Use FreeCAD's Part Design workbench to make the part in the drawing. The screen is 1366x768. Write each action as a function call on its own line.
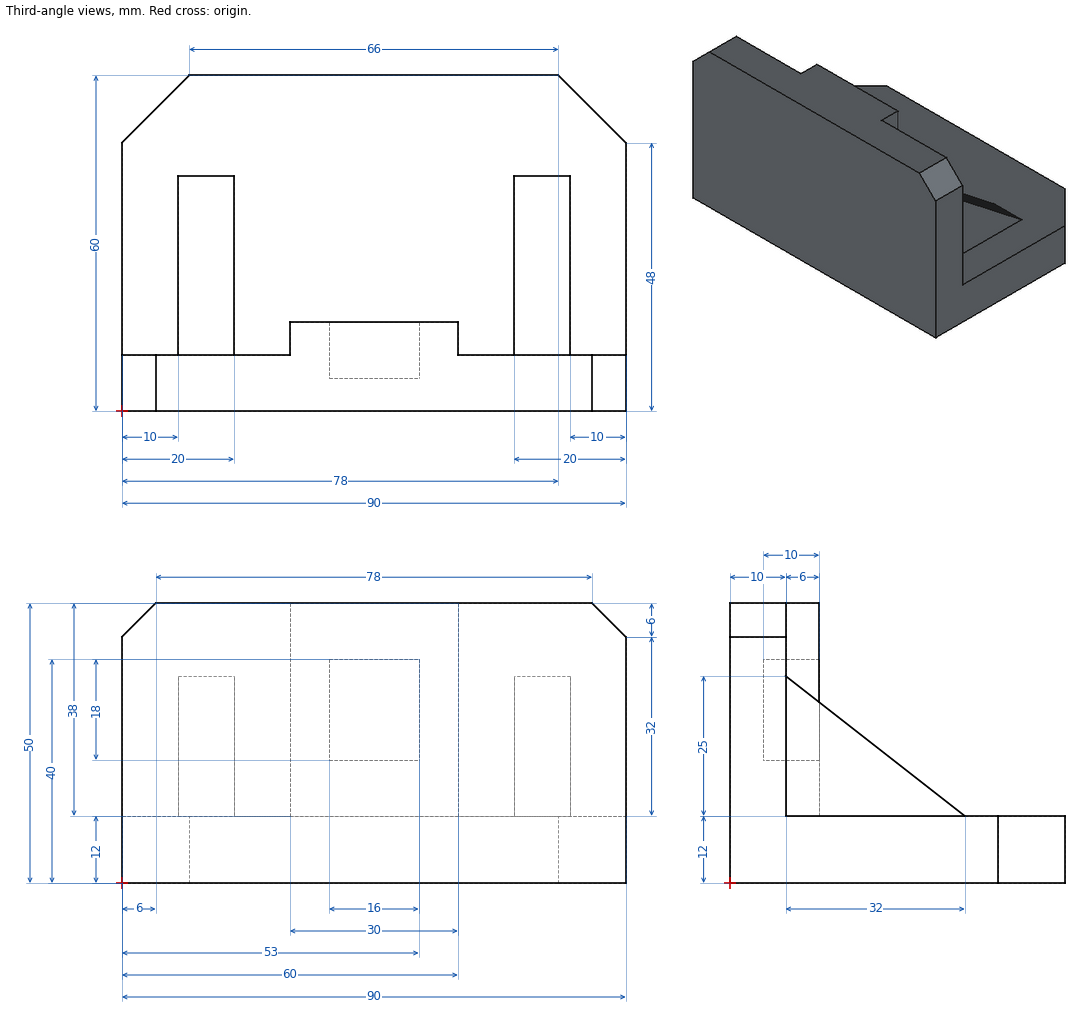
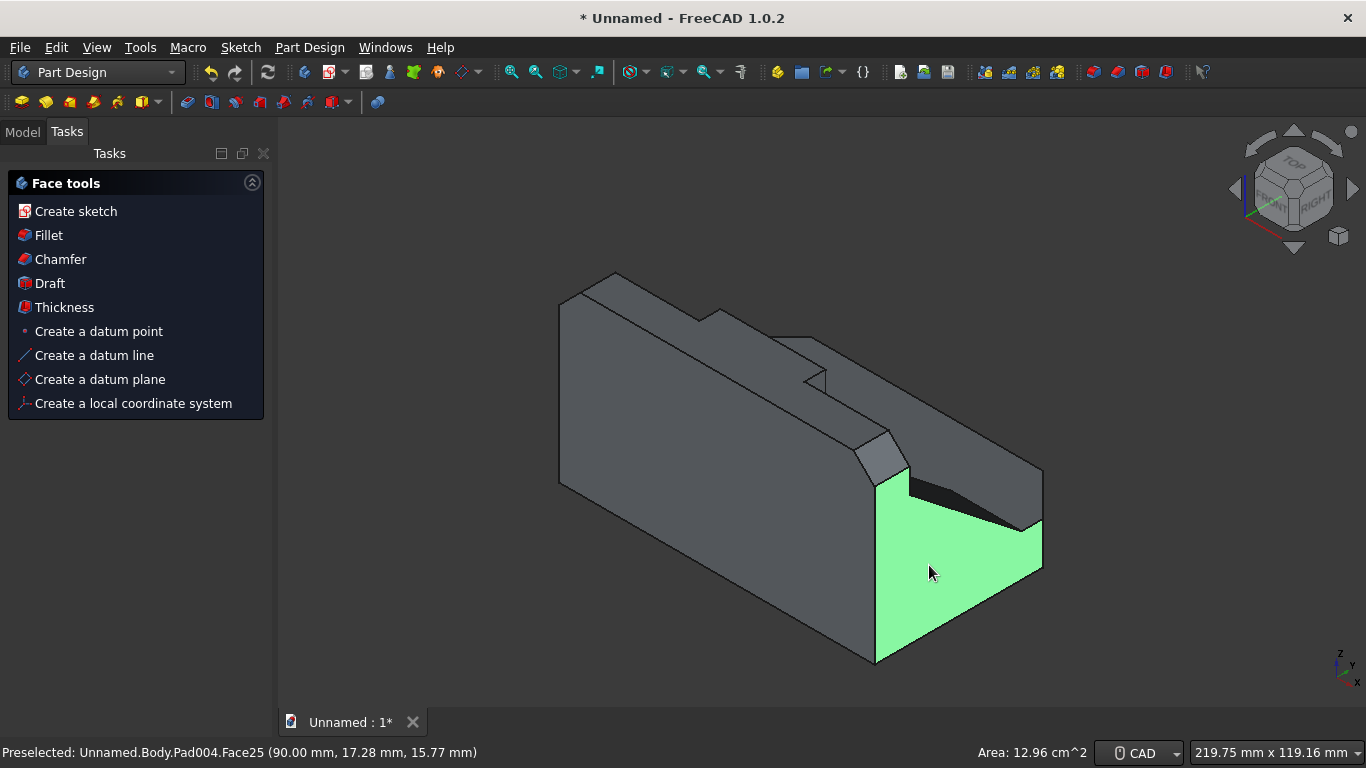
click(330, 72)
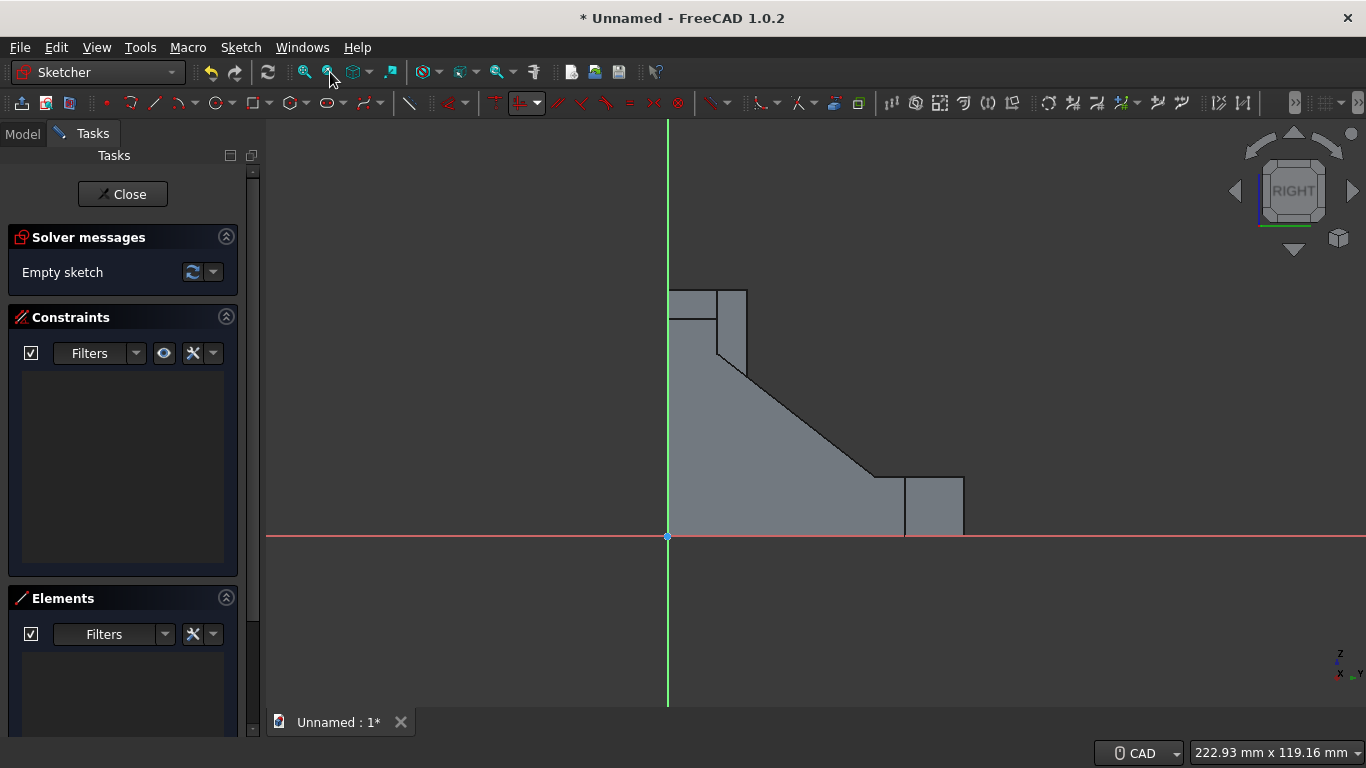
scroll(791, 471, up, 4)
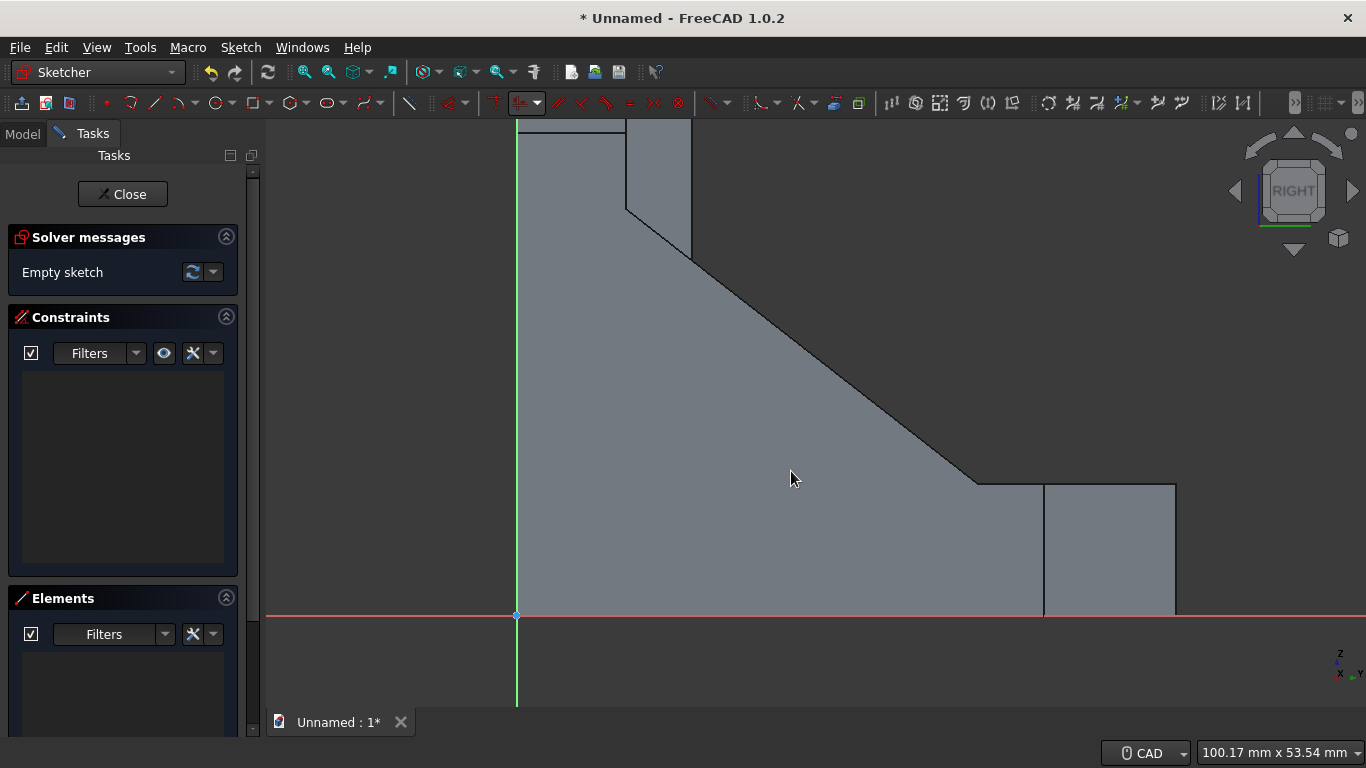
click(132, 104)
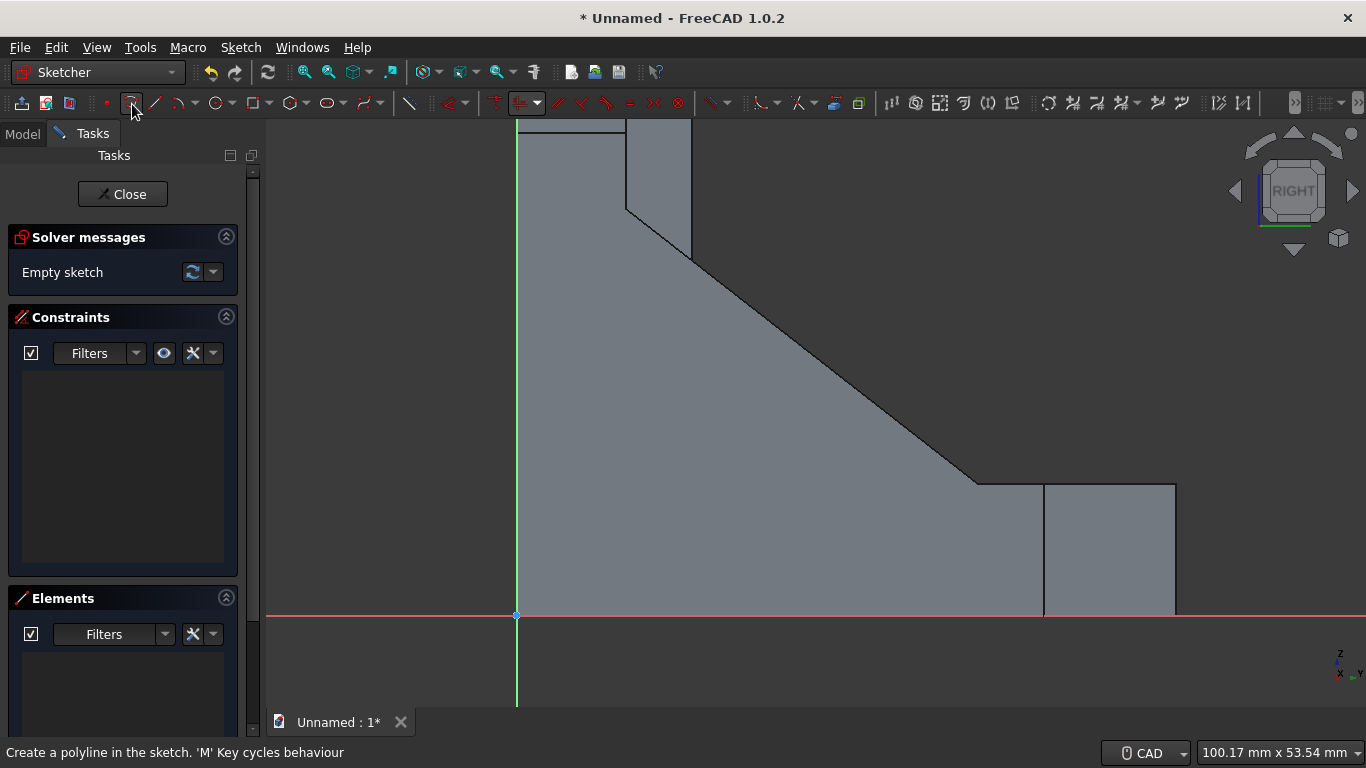
click(626, 484)
click(978, 484)
click(626, 209)
click(626, 485)
key(Escape)
key(Escape)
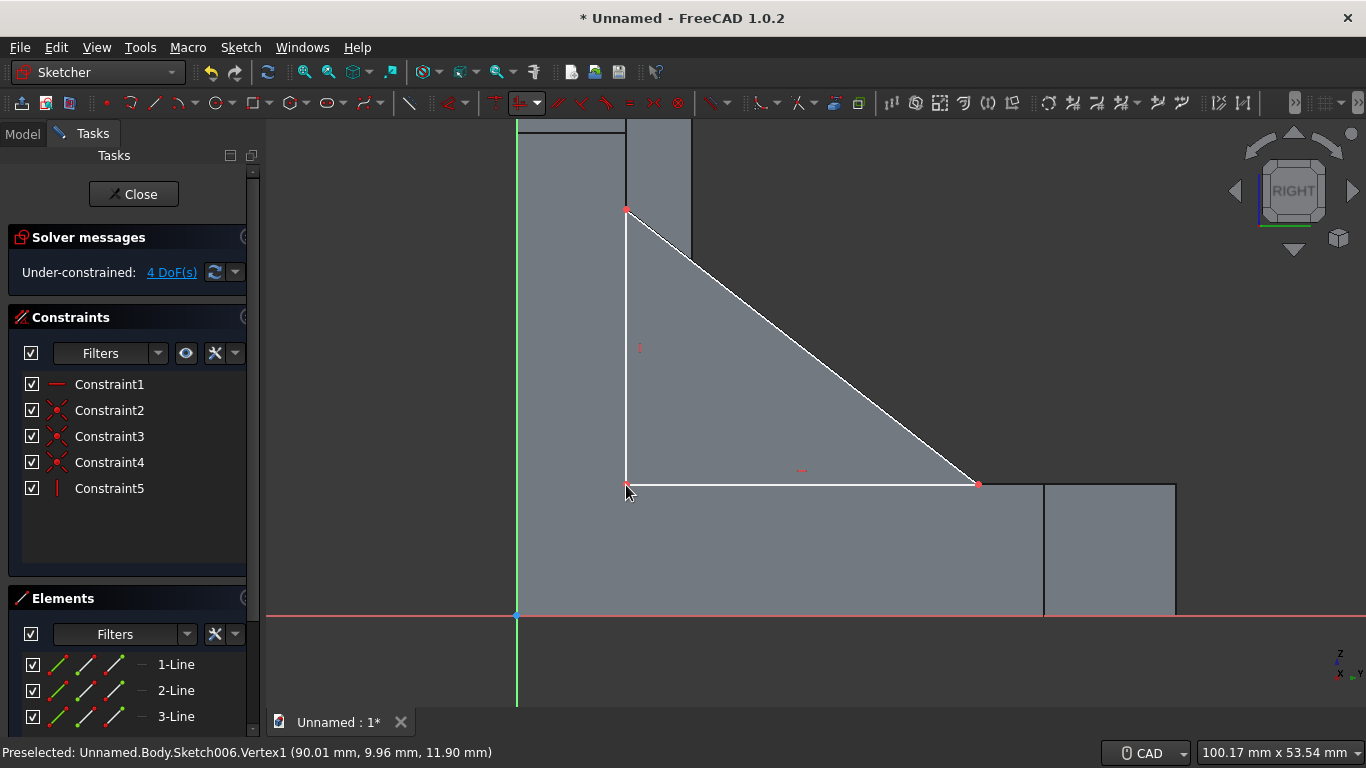
click(448, 104)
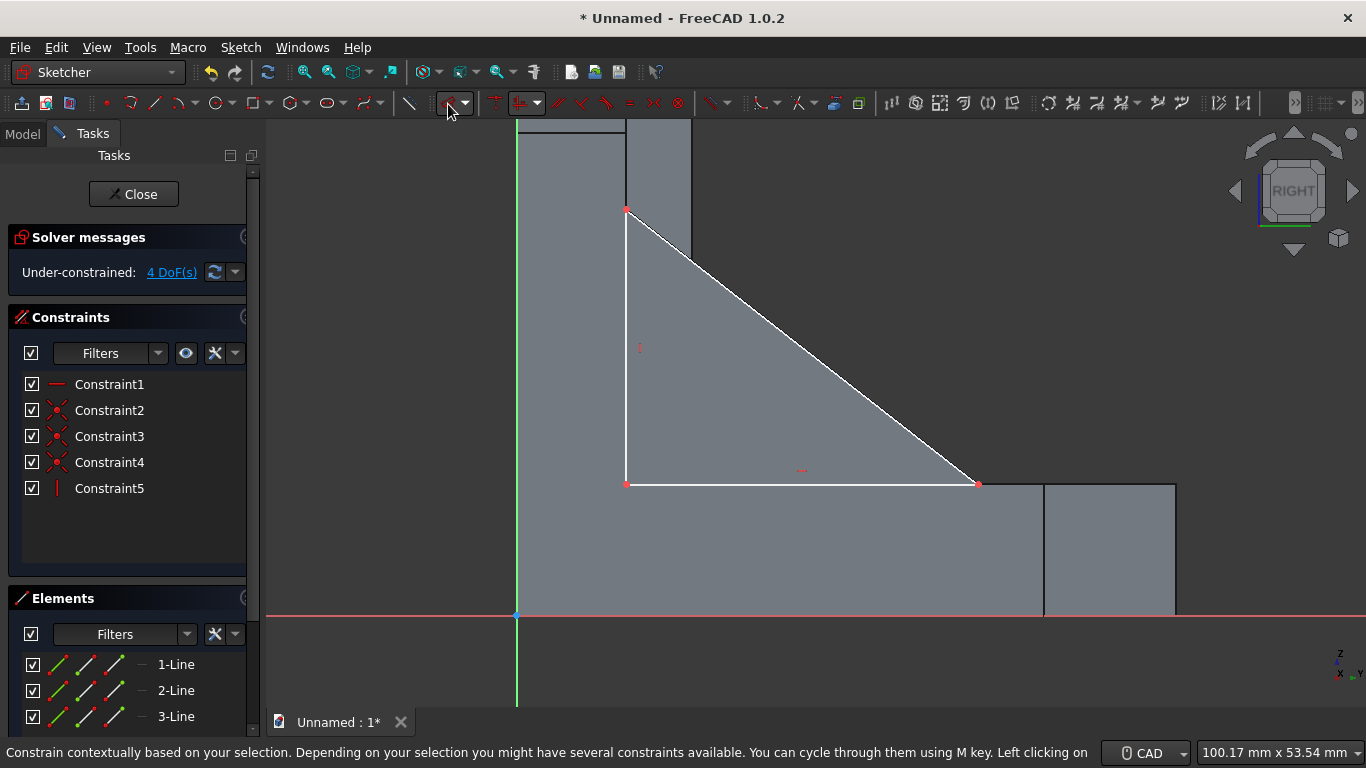
click(732, 485)
click(802, 519)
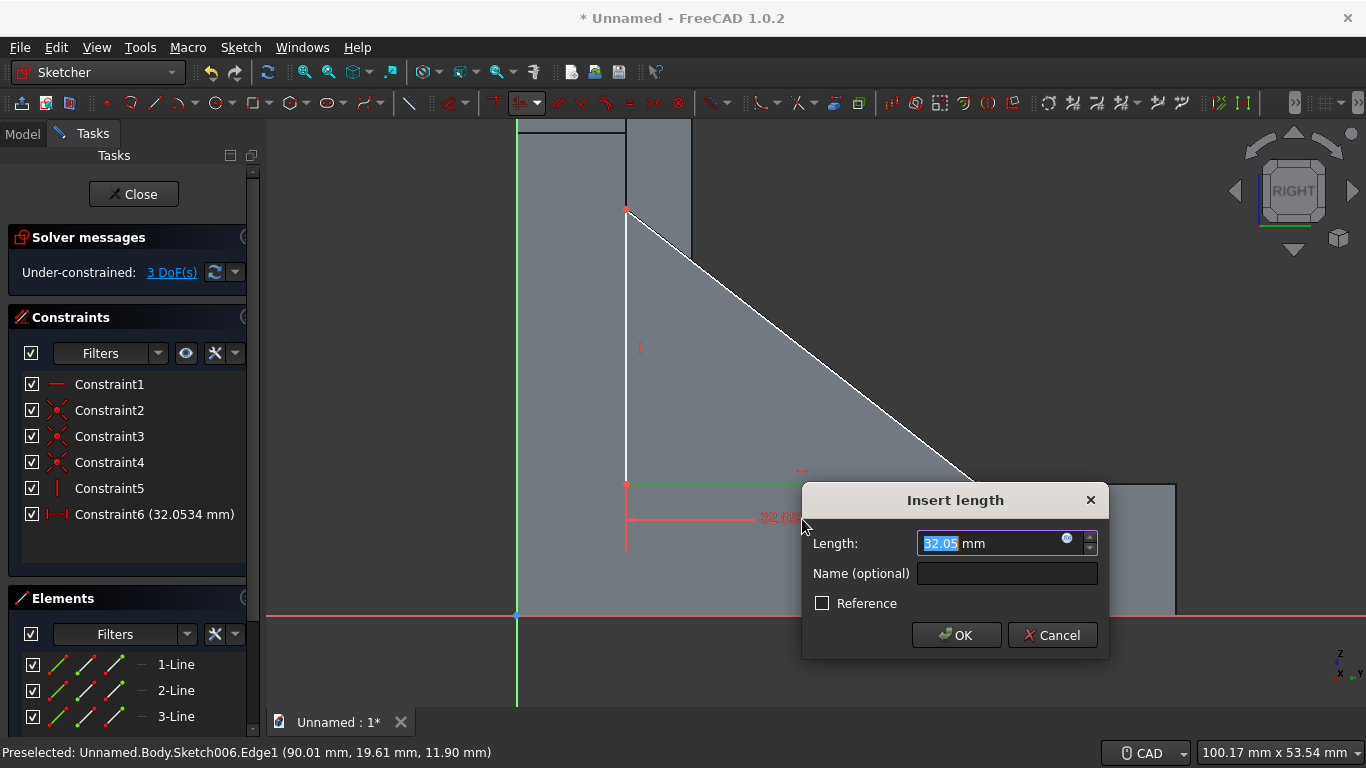
text(32)
key(Return)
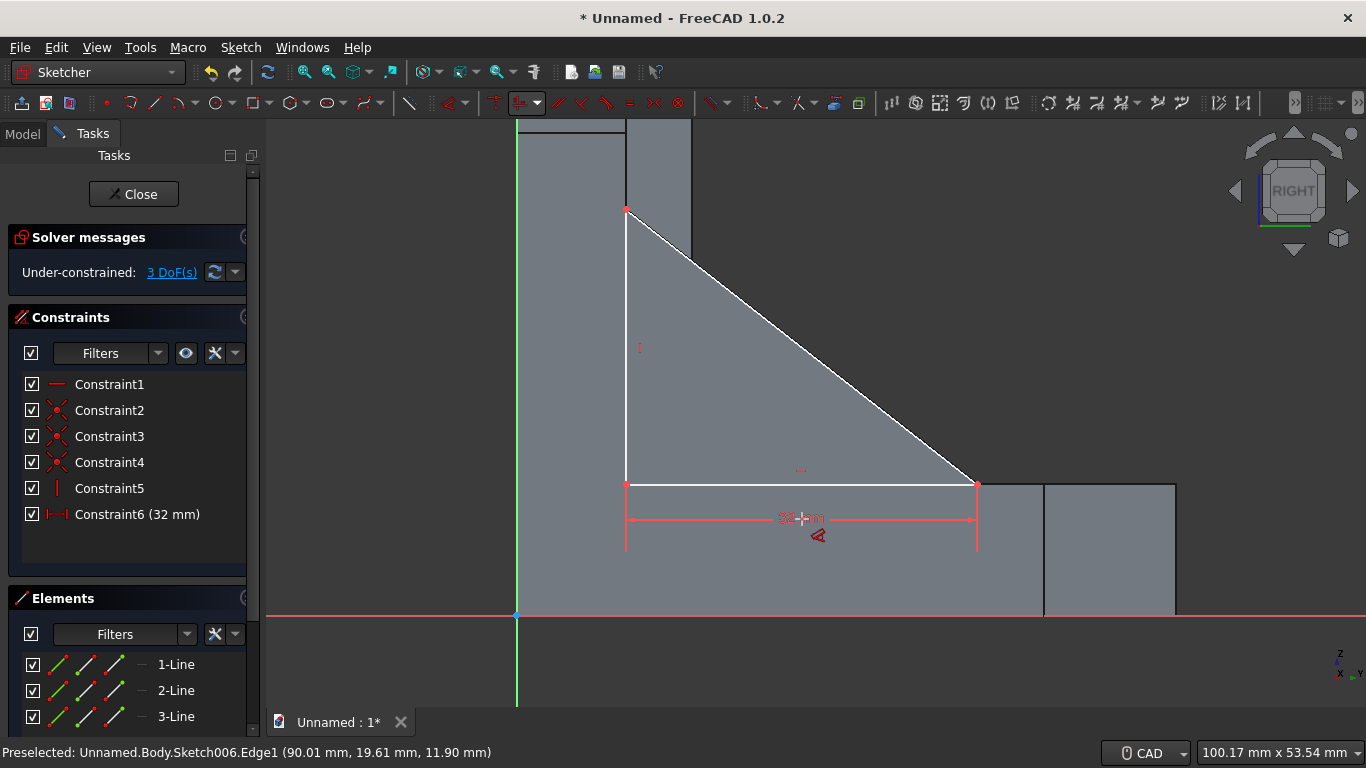
click(626, 292)
click(592, 347)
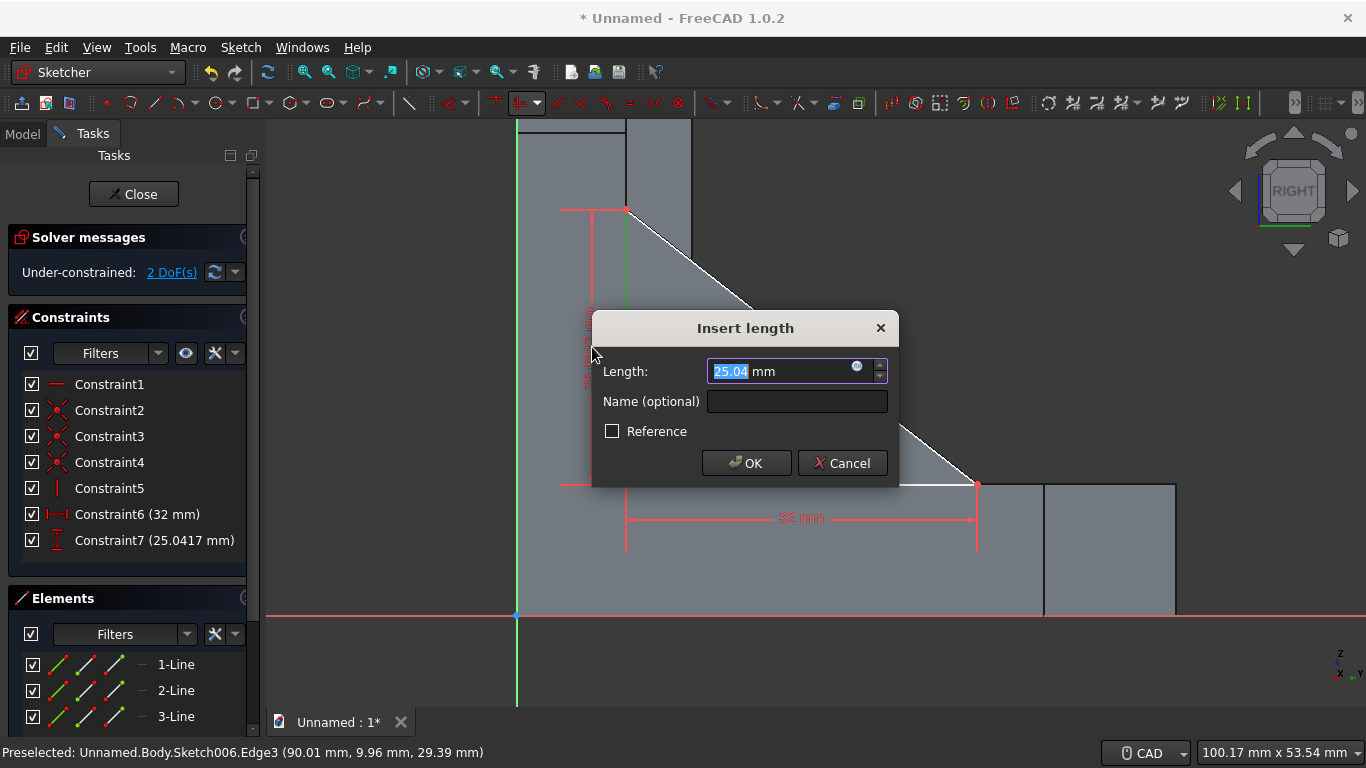
text(25)
key(Return)